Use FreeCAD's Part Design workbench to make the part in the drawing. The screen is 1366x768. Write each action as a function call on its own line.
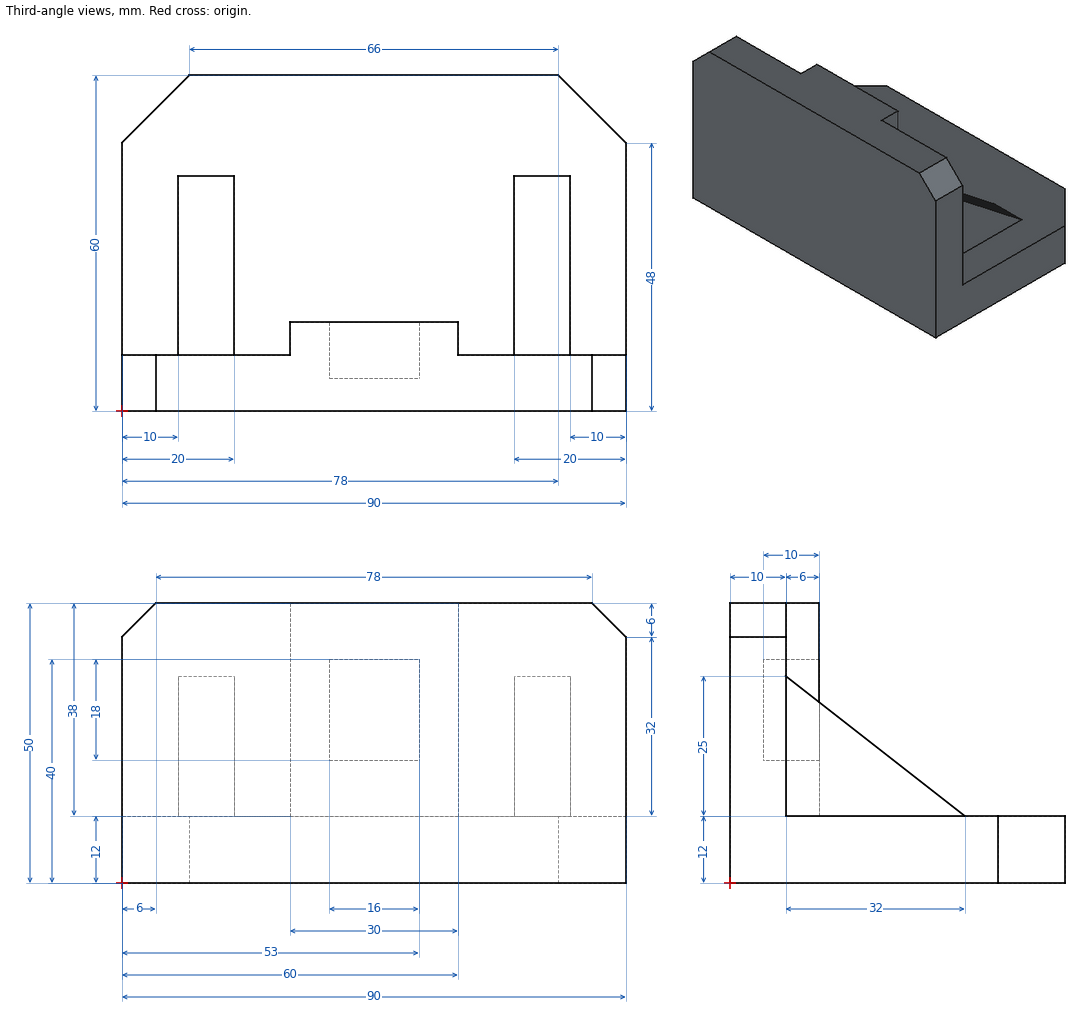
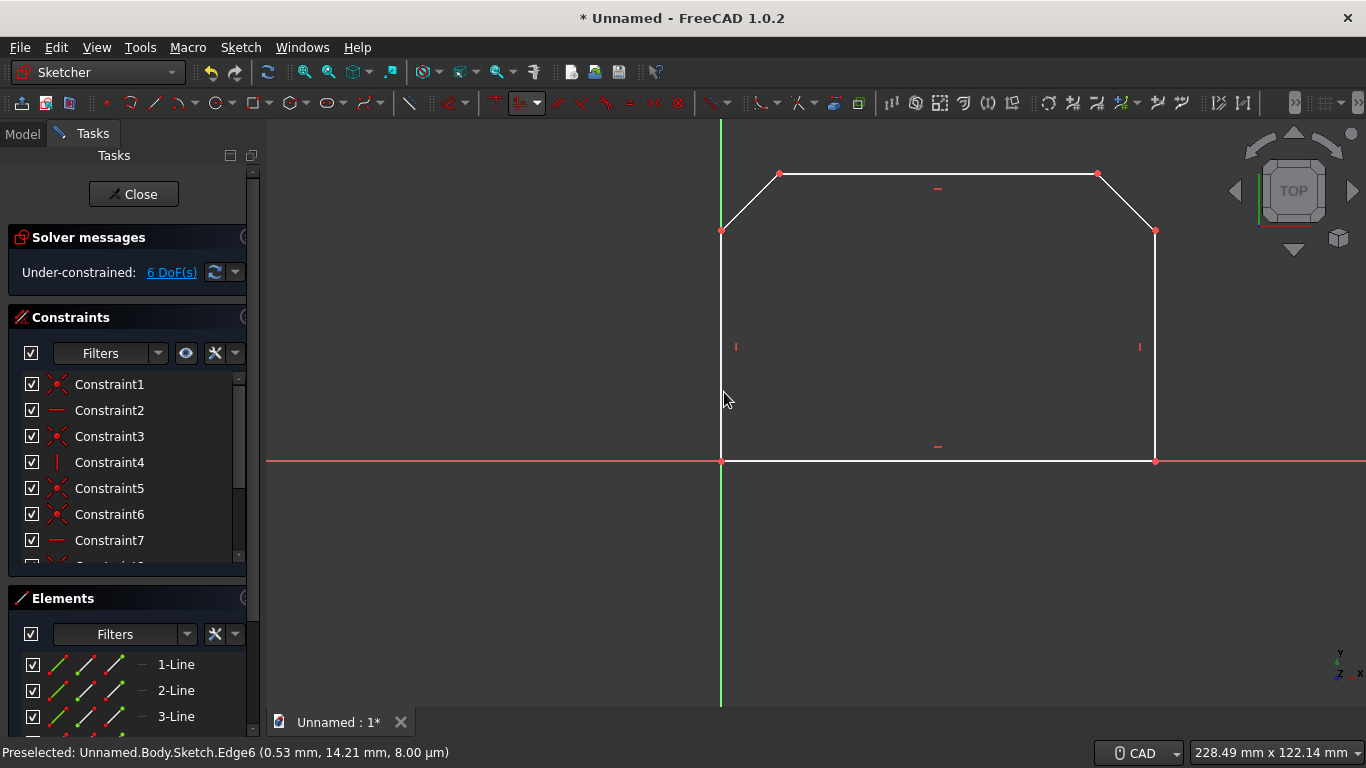
click(448, 104)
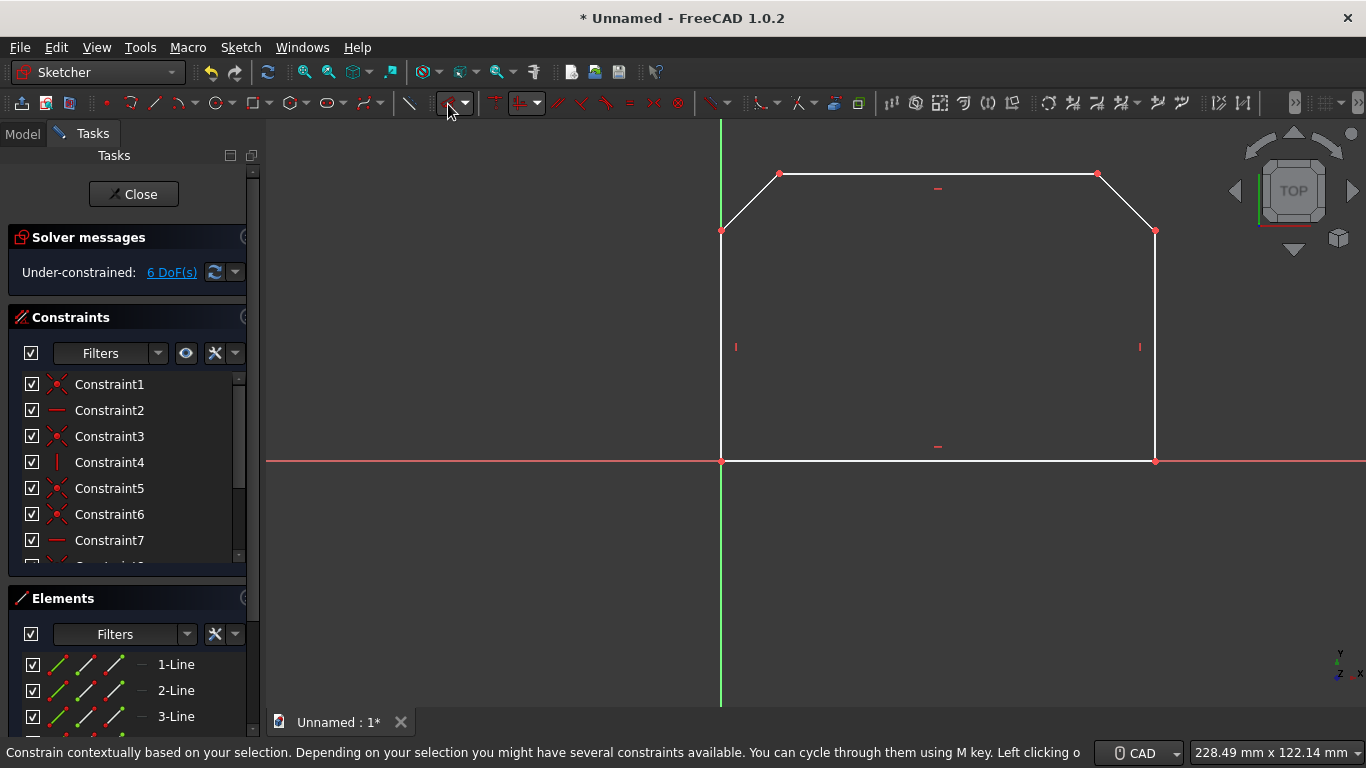
click(851, 461)
click(938, 495)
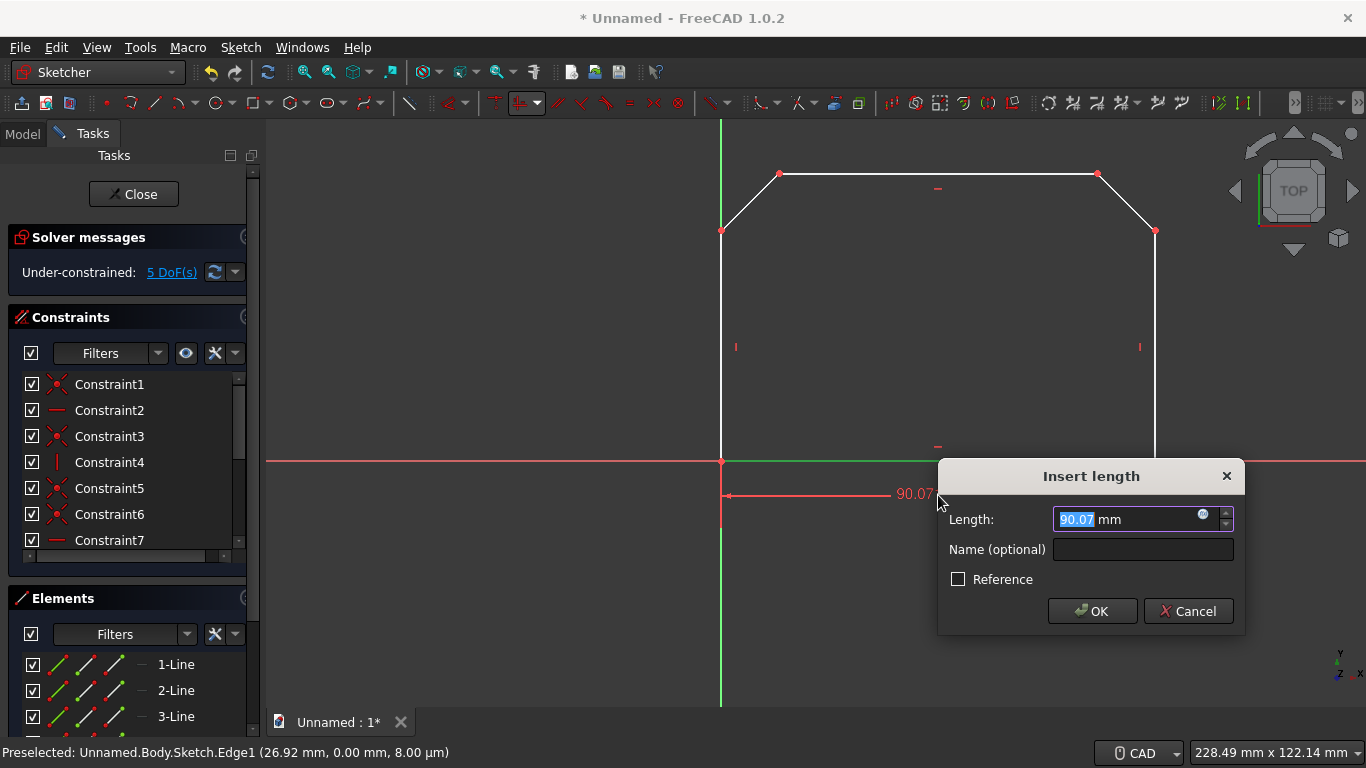
text(90)
key(Return)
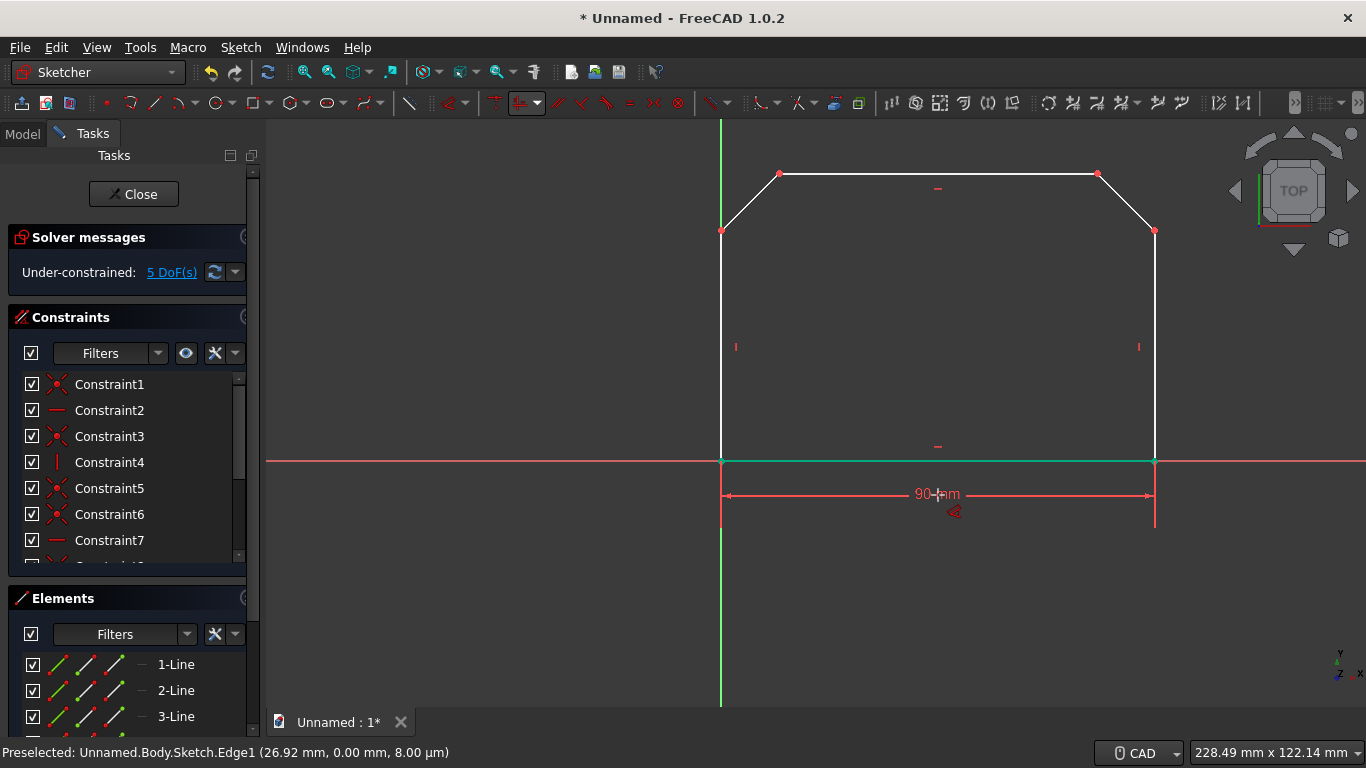
click(1155, 392)
click(1189, 346)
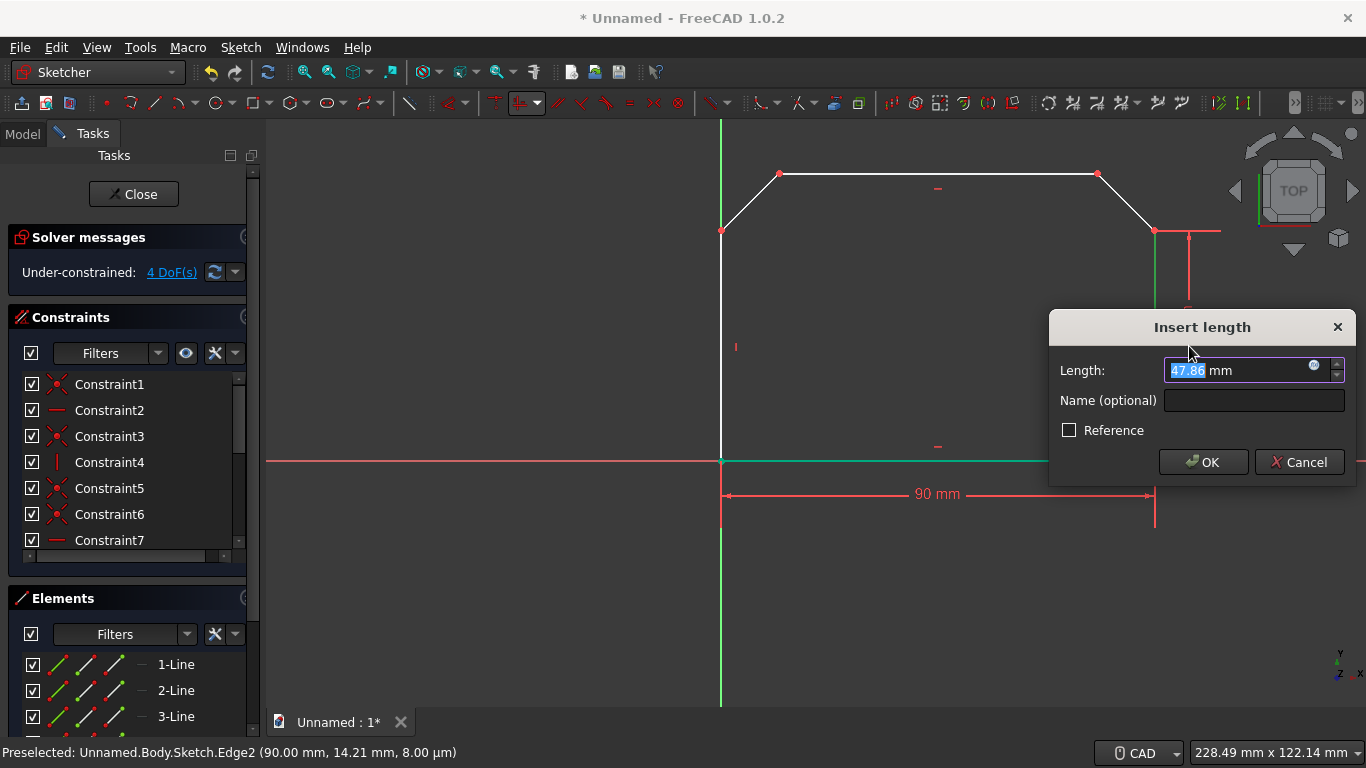
text(48)
key(Return)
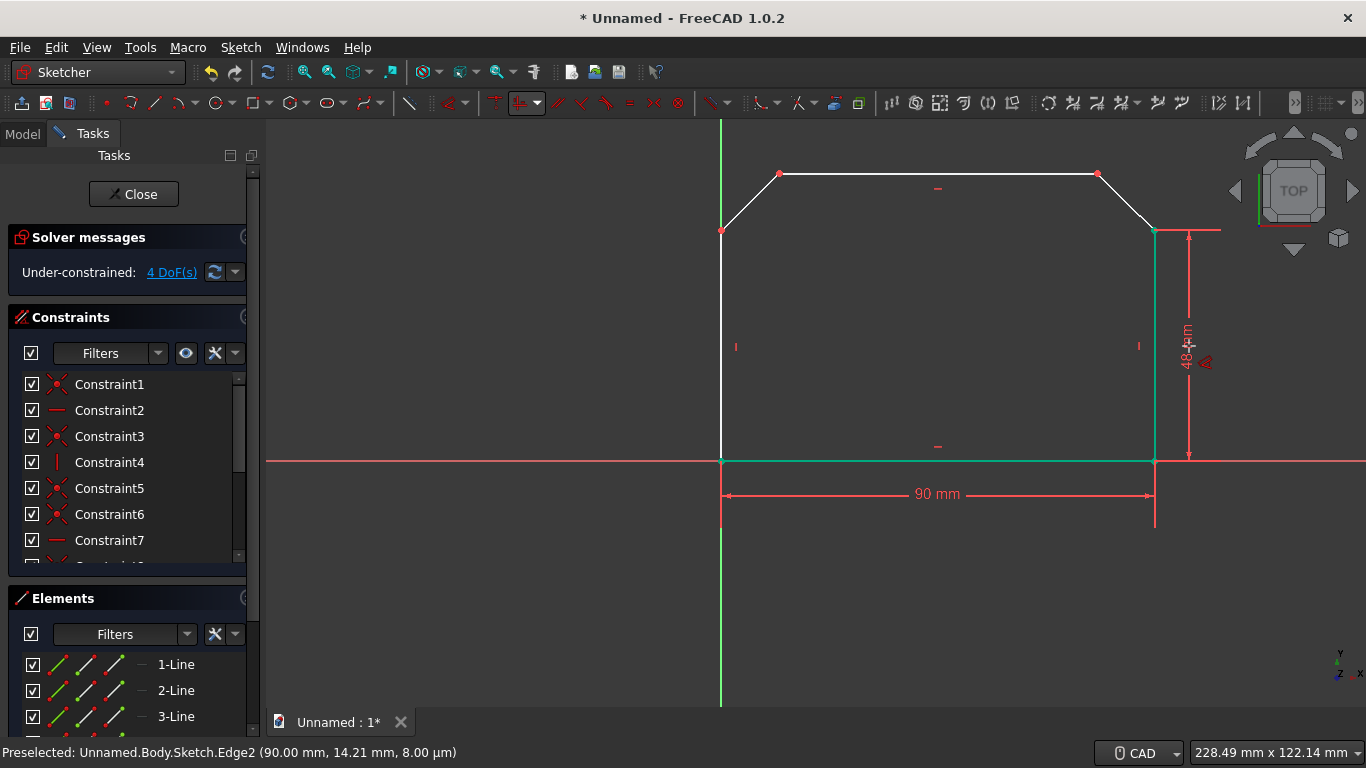
click(1002, 174)
click(938, 208)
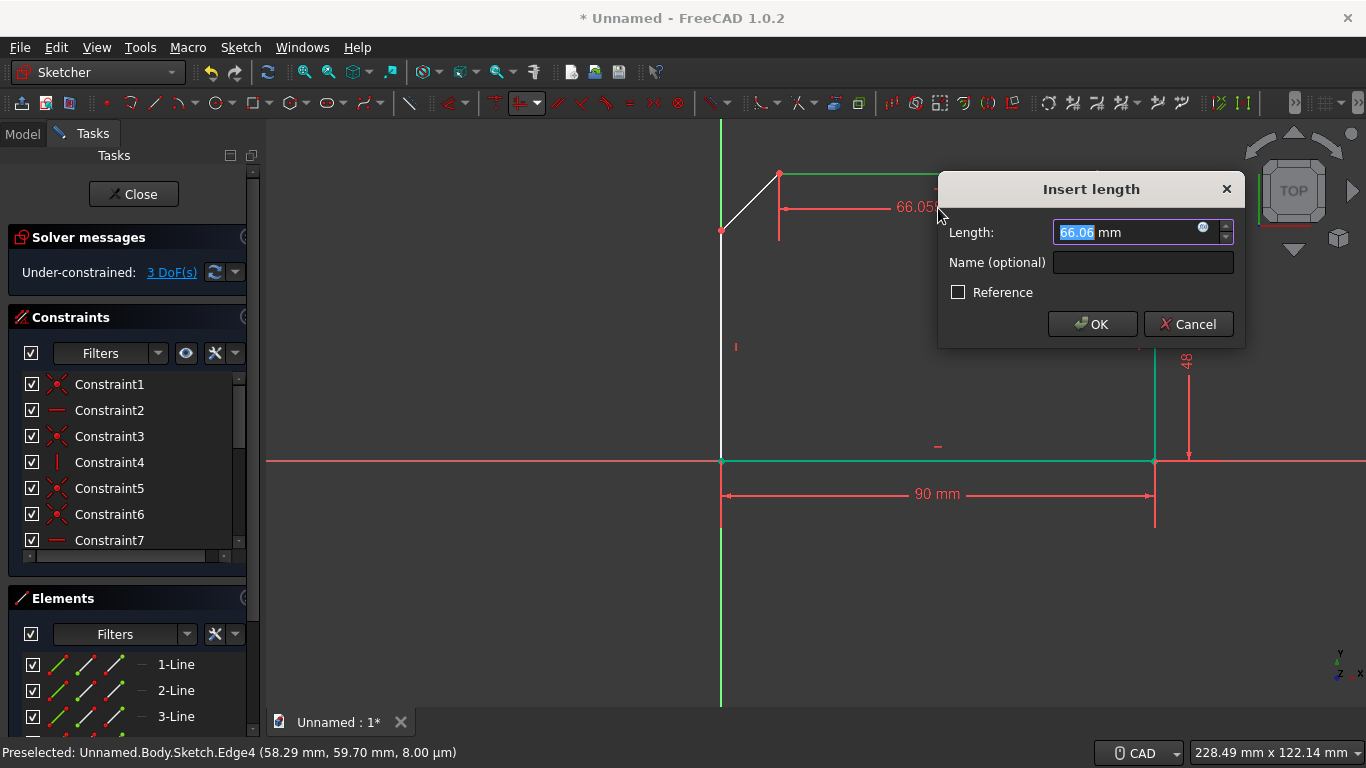
text(66)
key(Return)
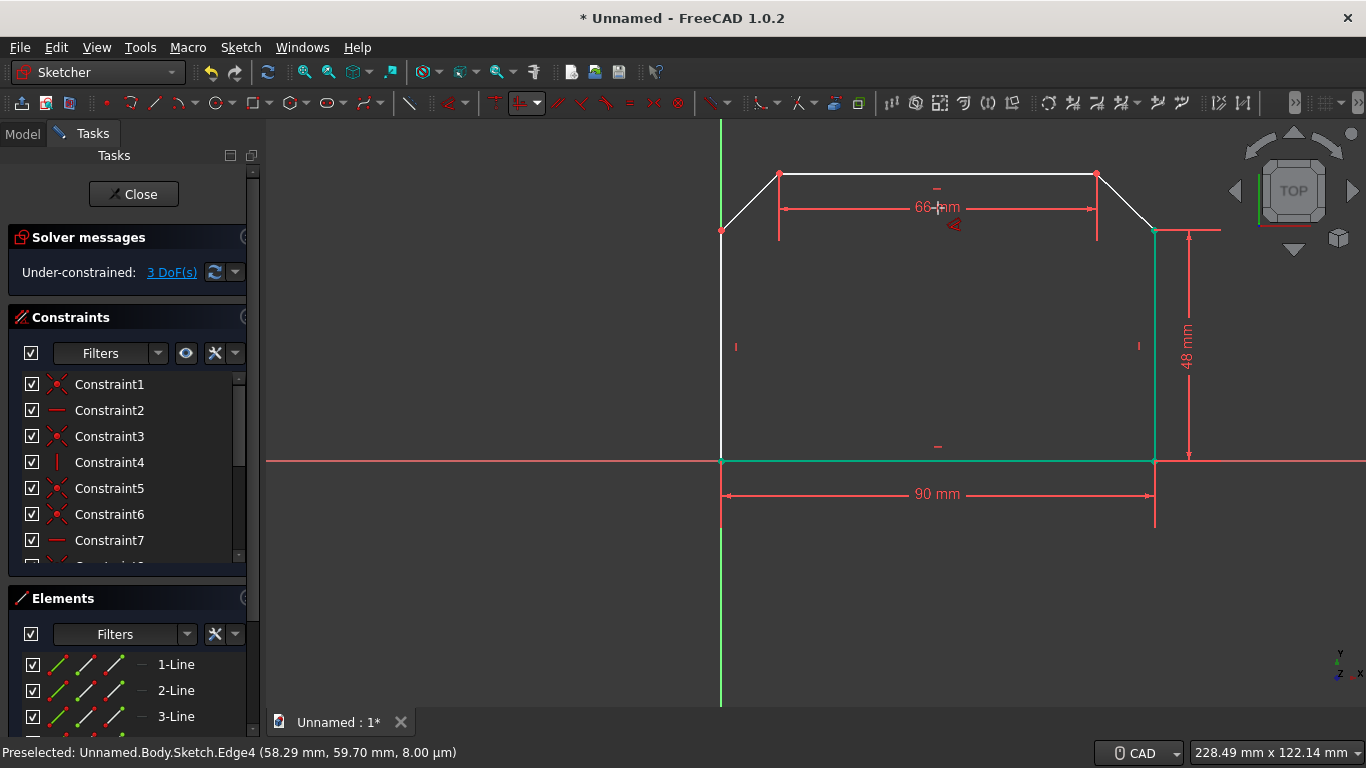
click(721, 300)
click(687, 346)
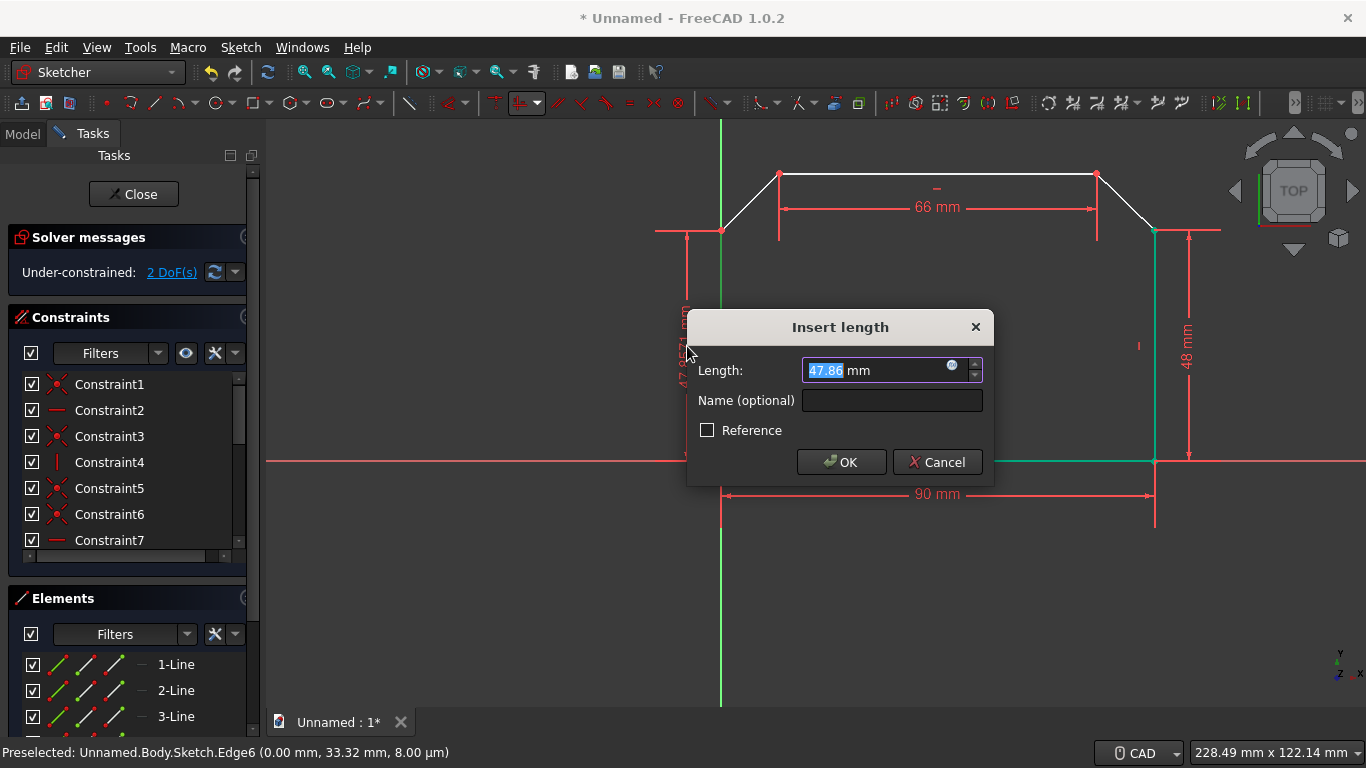
text(48)
key(Return)